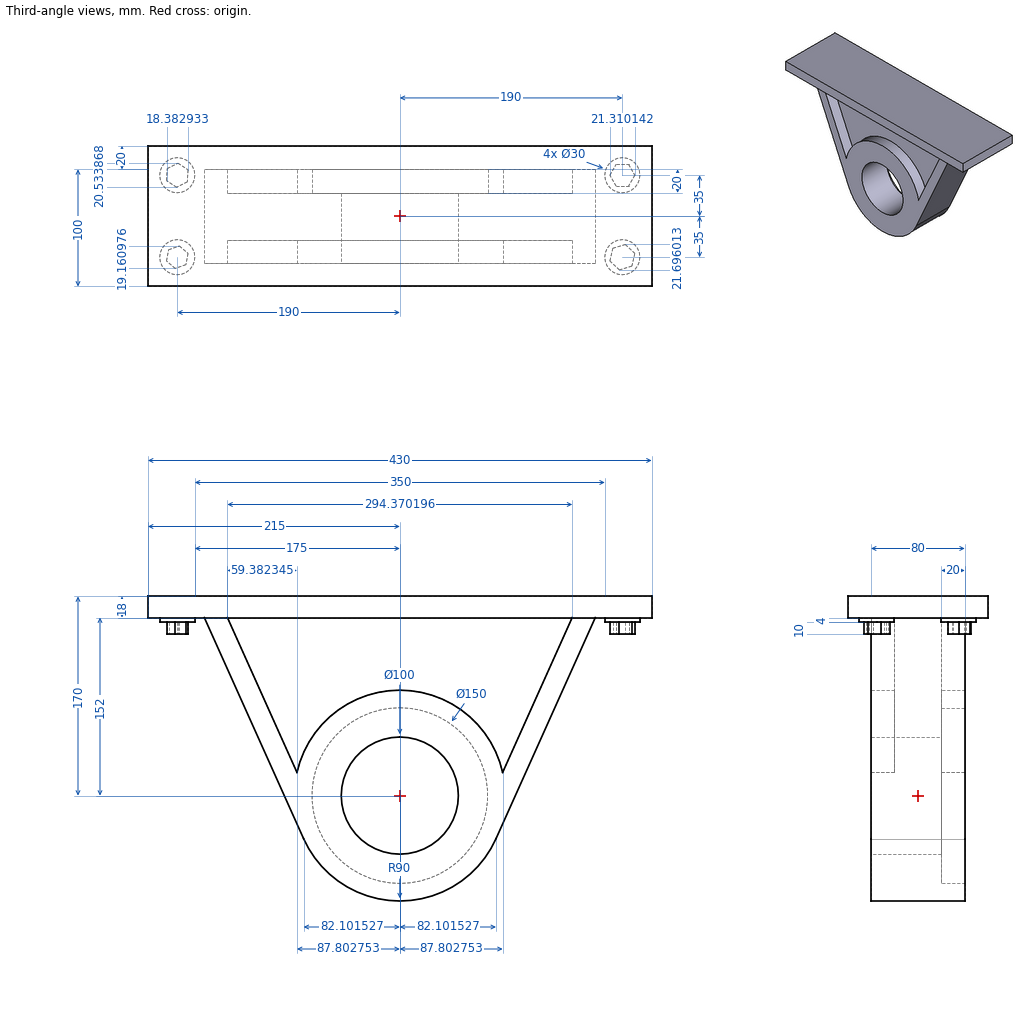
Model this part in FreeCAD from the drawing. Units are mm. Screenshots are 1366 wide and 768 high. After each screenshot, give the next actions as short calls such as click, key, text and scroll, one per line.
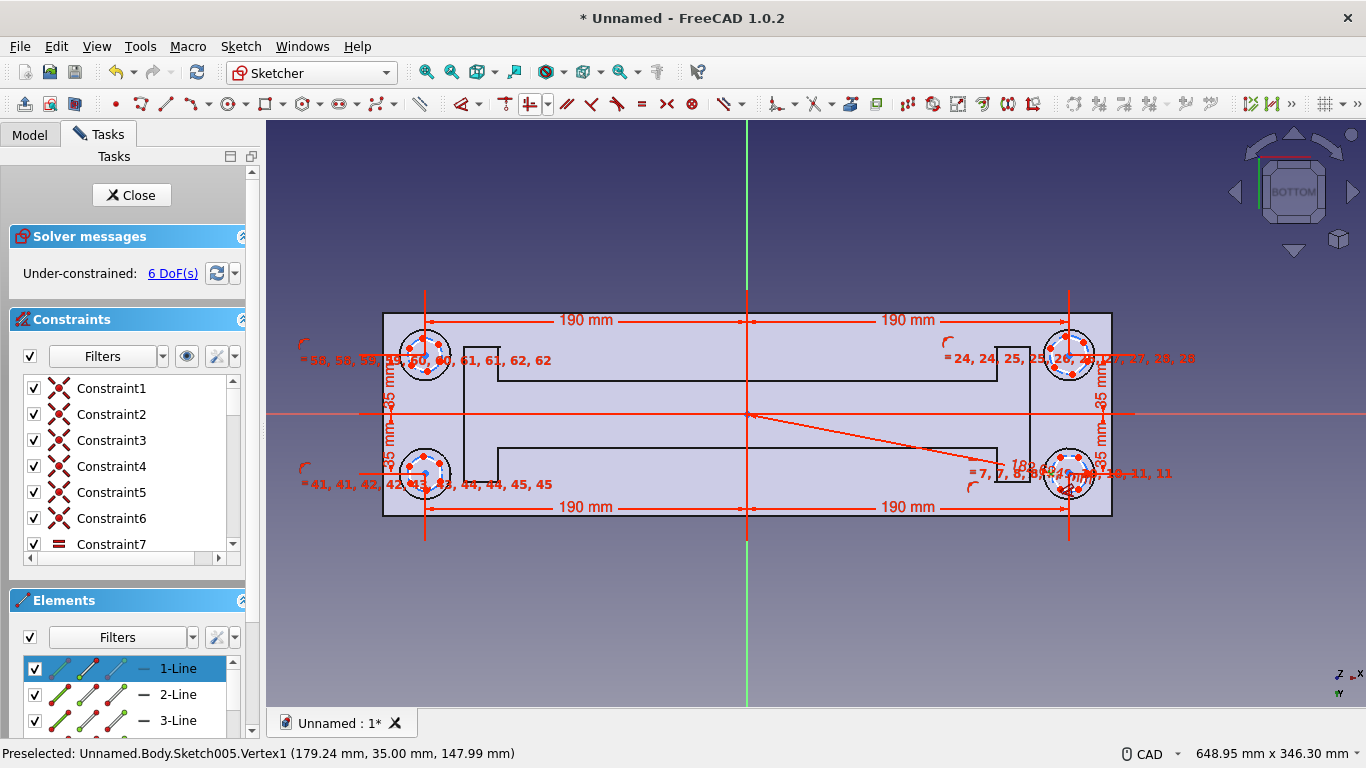
click(1087, 474)
click(1069, 508)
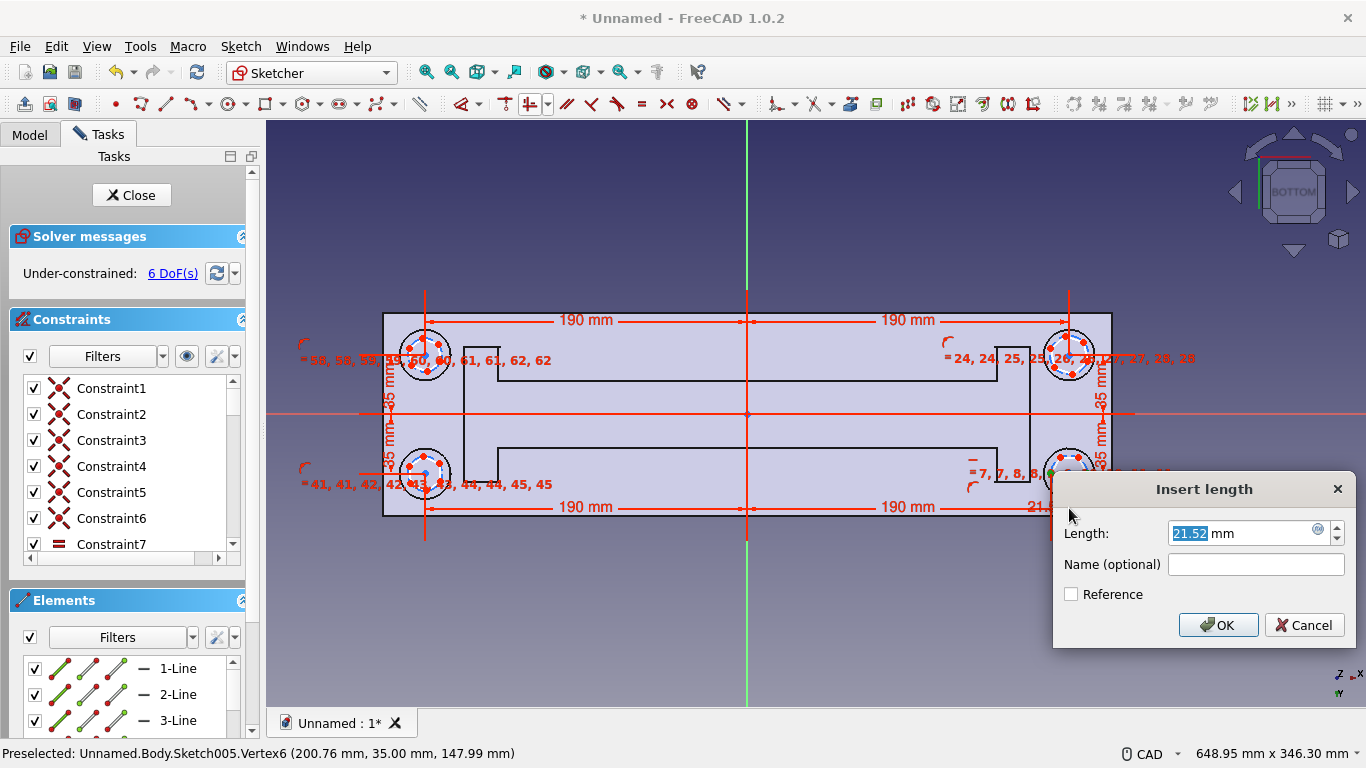
text(21.310142)
key(Return)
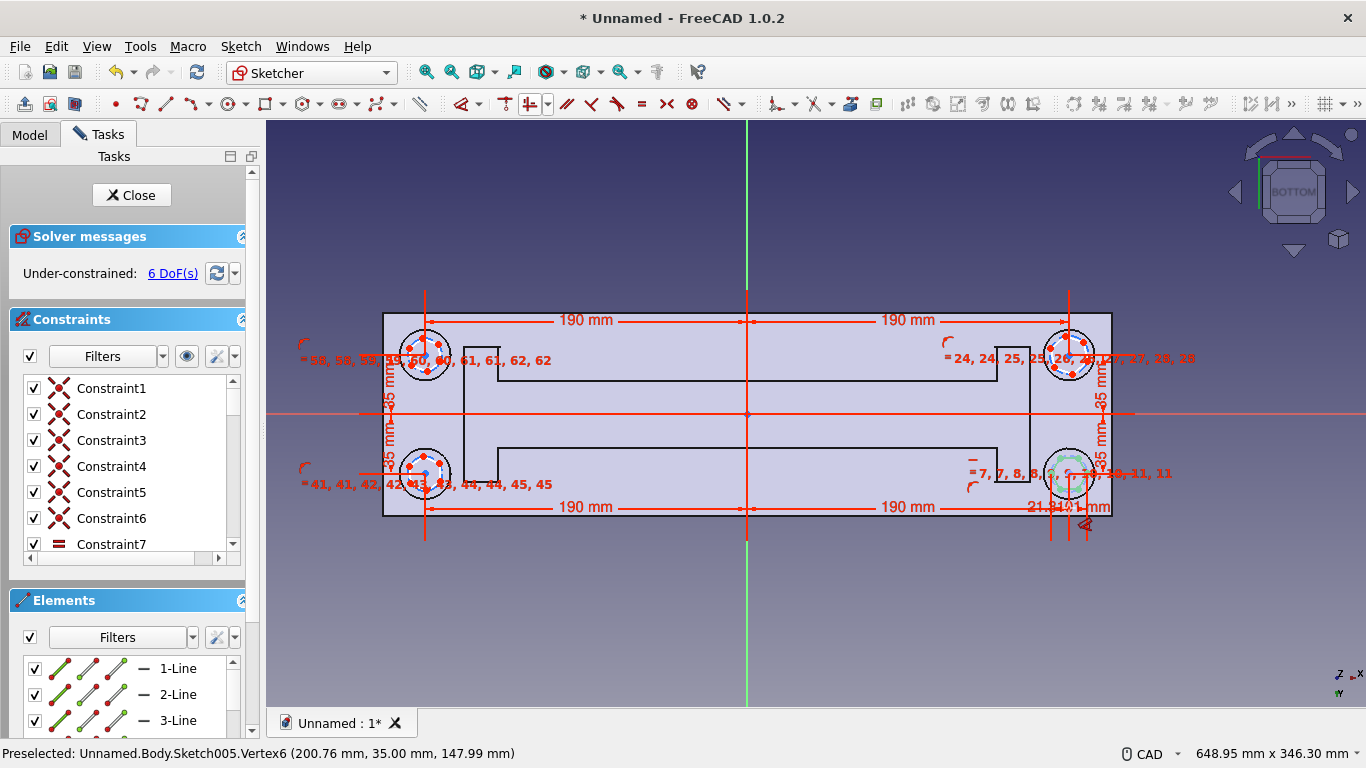
click(1051, 349)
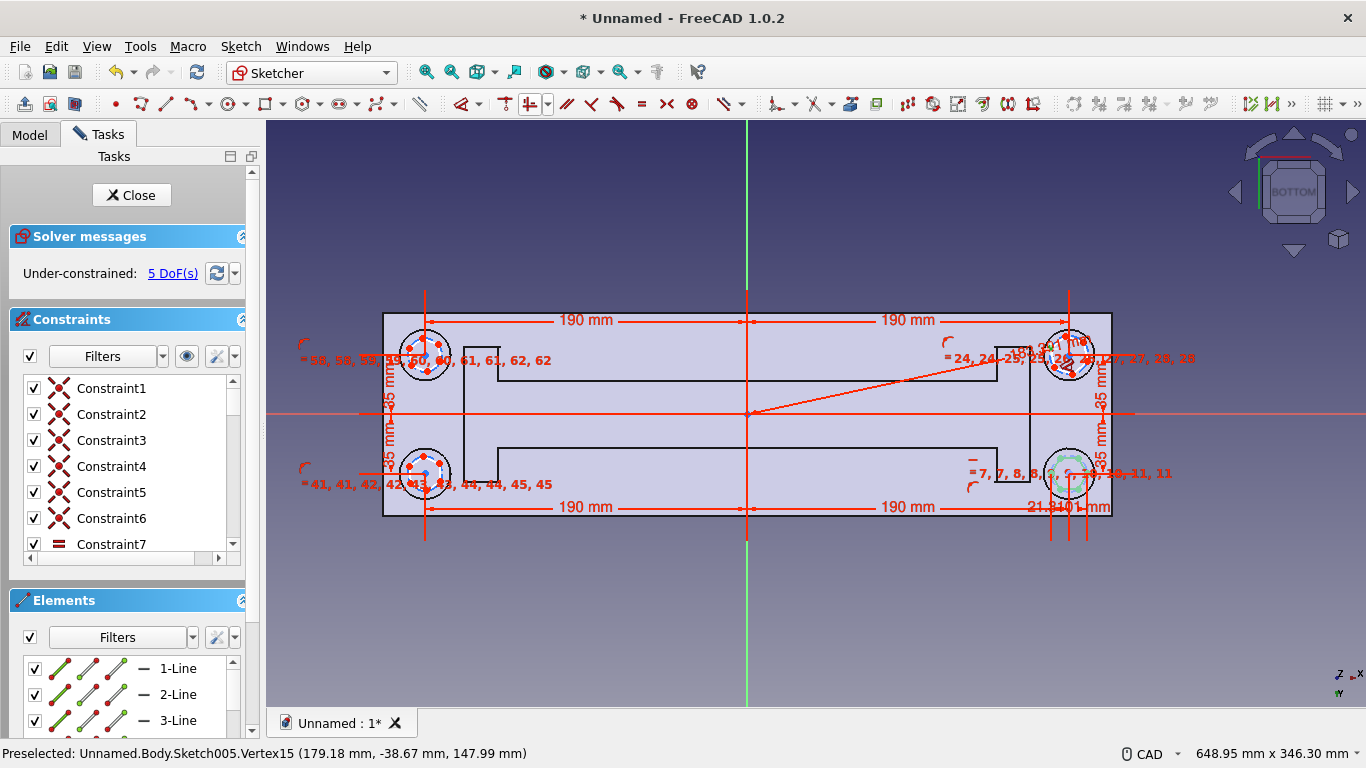
click(1088, 361)
click(1069, 315)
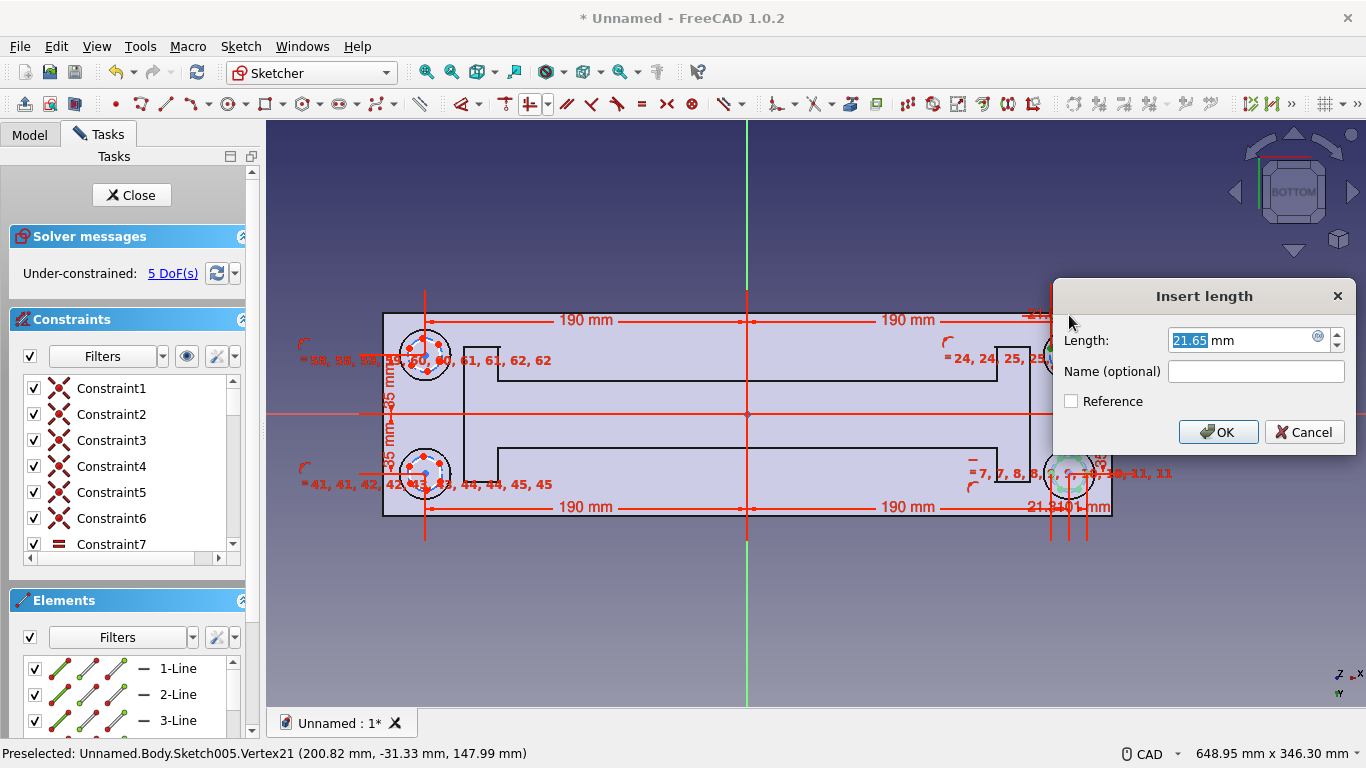
text(21.310142)
key(Return)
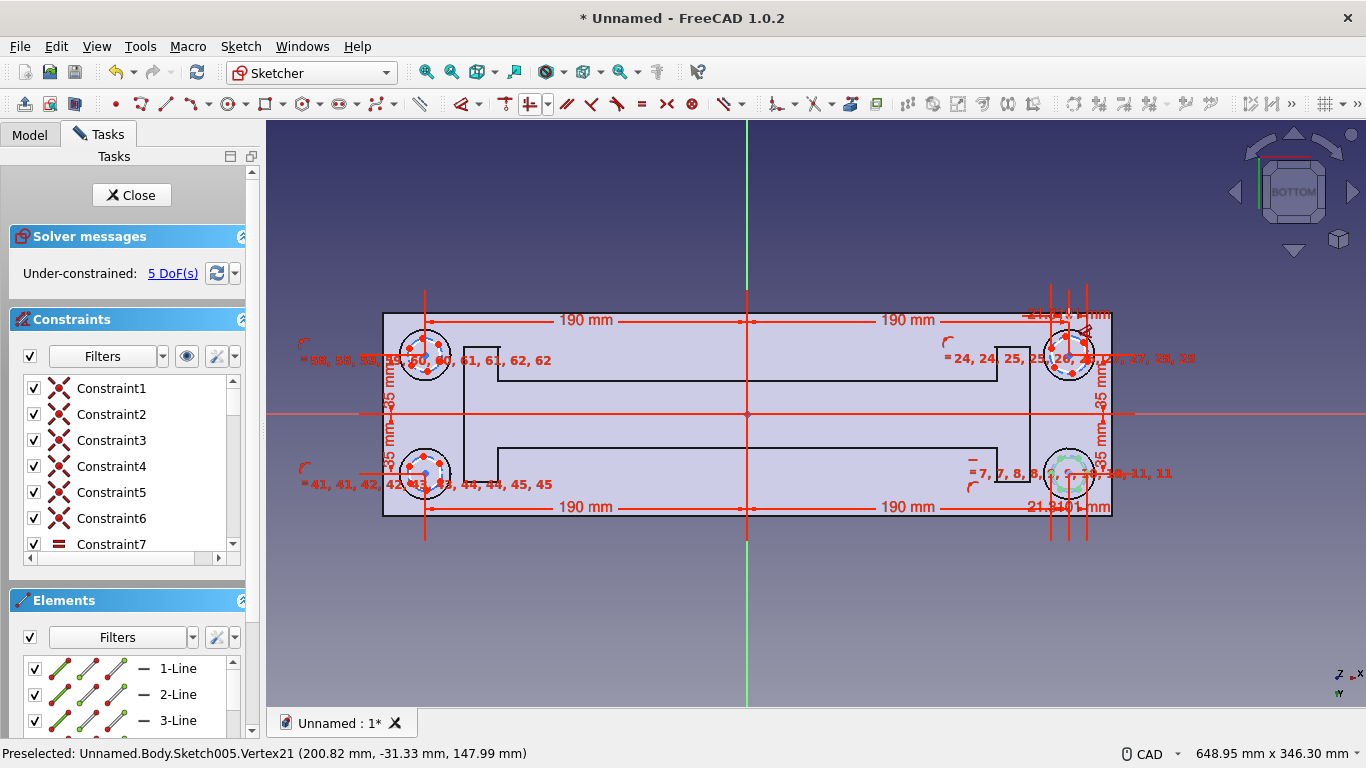
click(1073, 374)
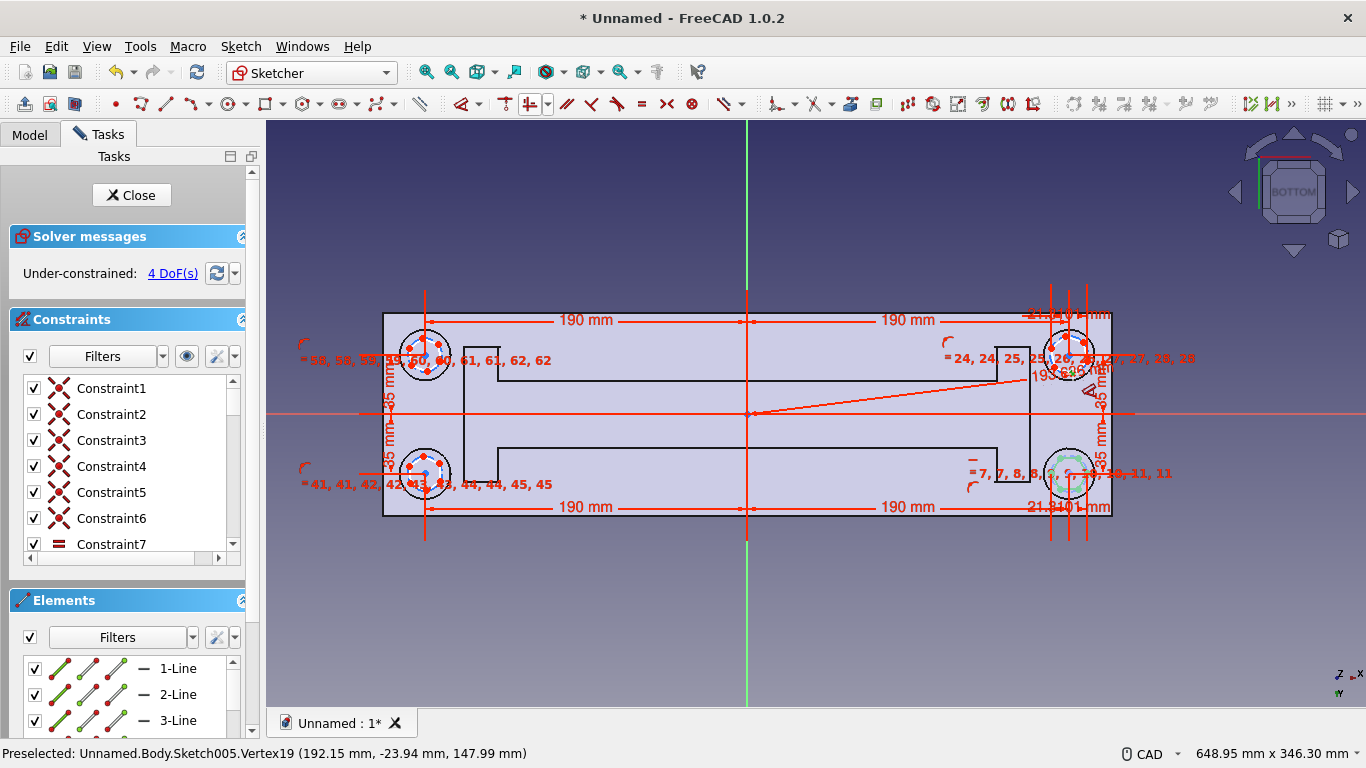
click(1066, 336)
click(1107, 355)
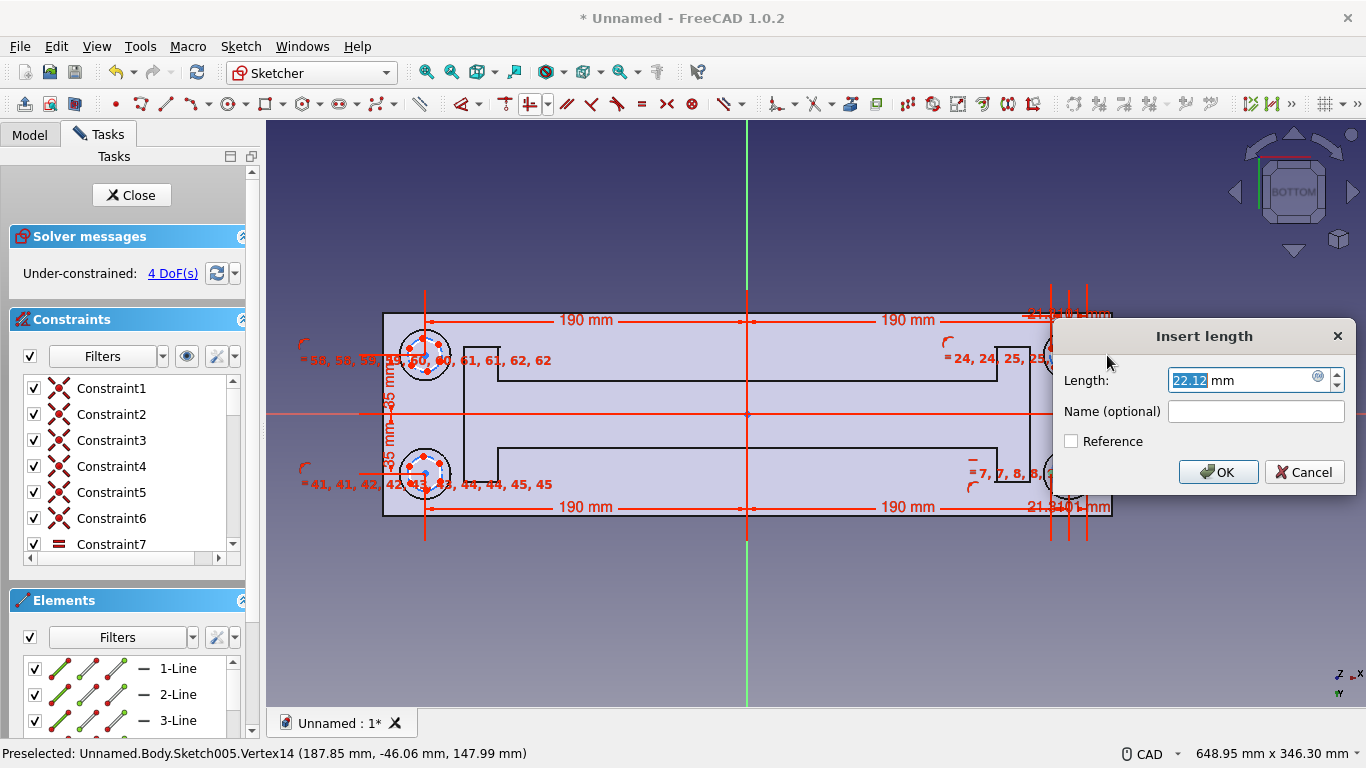
text(21.696013)
key(Return)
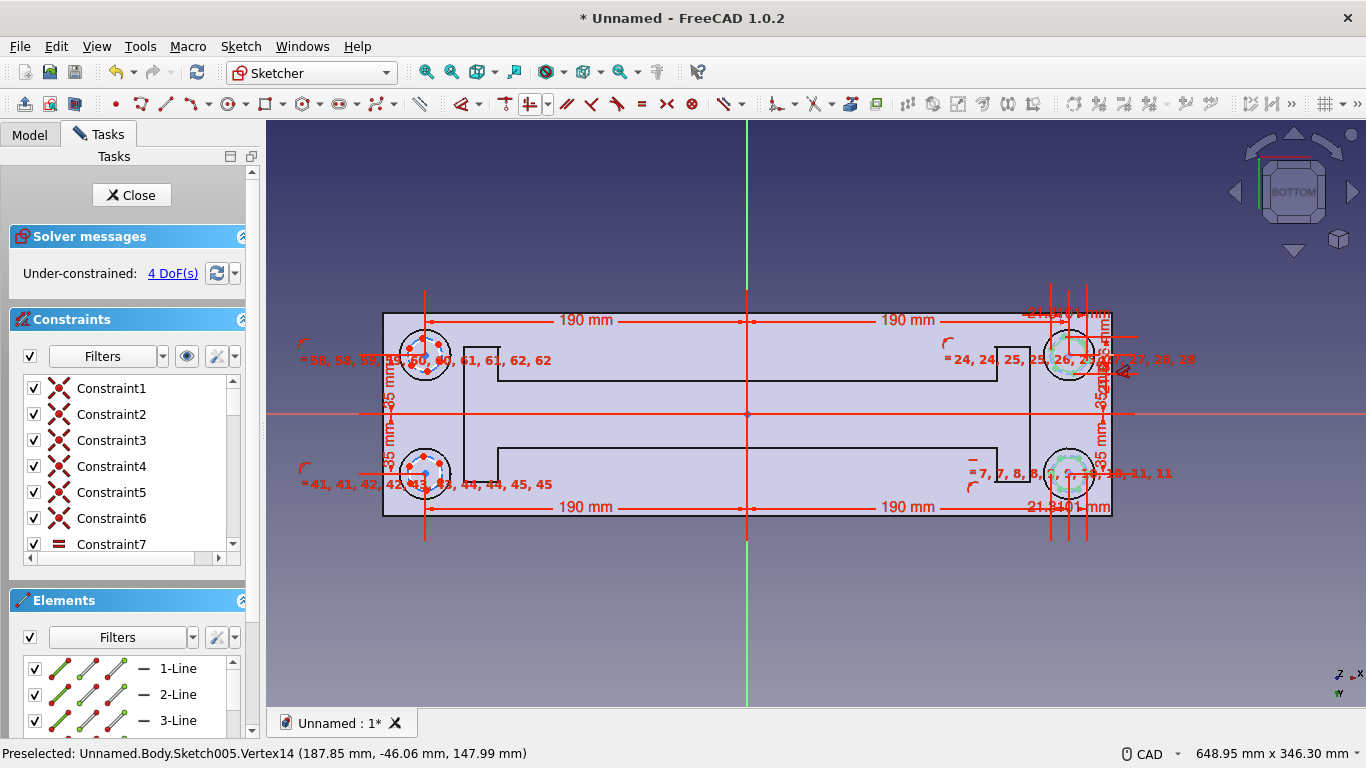
scroll(409, 466, up, 2)